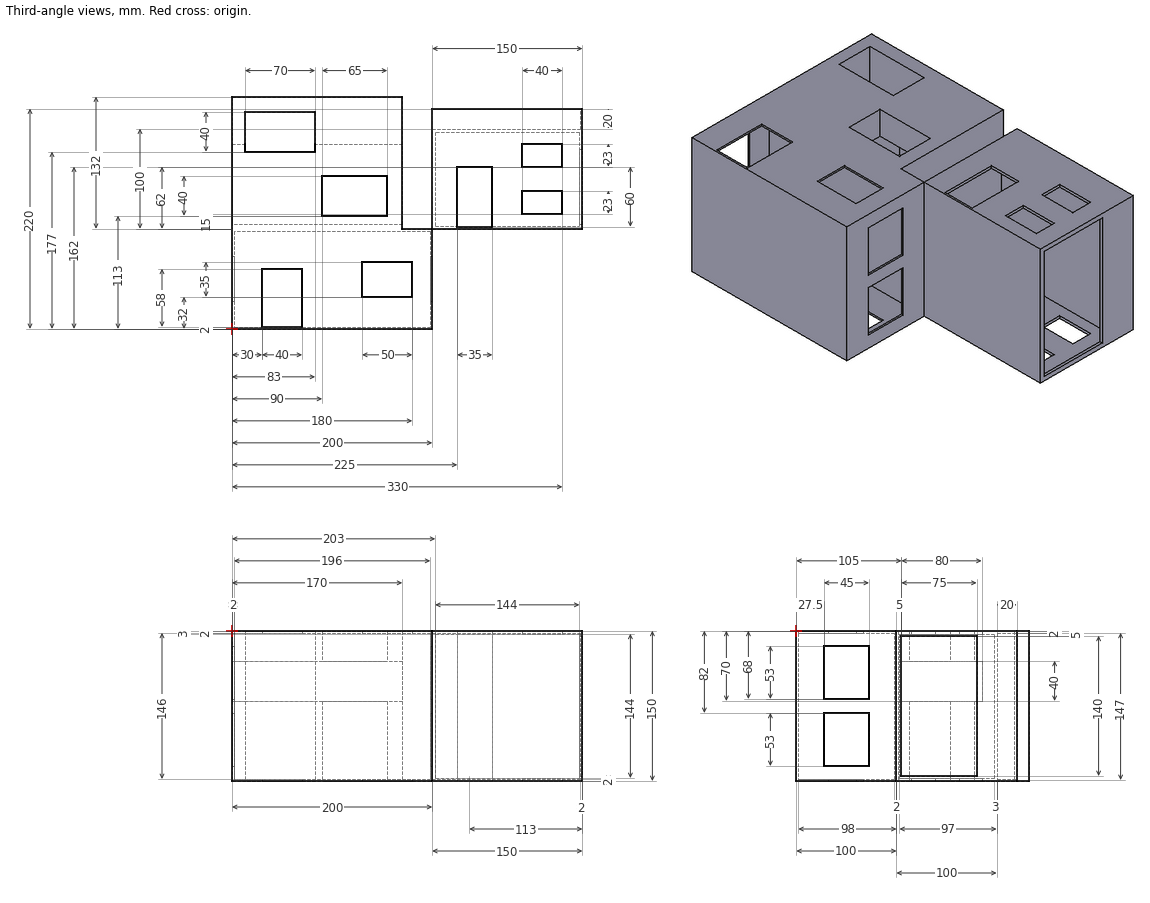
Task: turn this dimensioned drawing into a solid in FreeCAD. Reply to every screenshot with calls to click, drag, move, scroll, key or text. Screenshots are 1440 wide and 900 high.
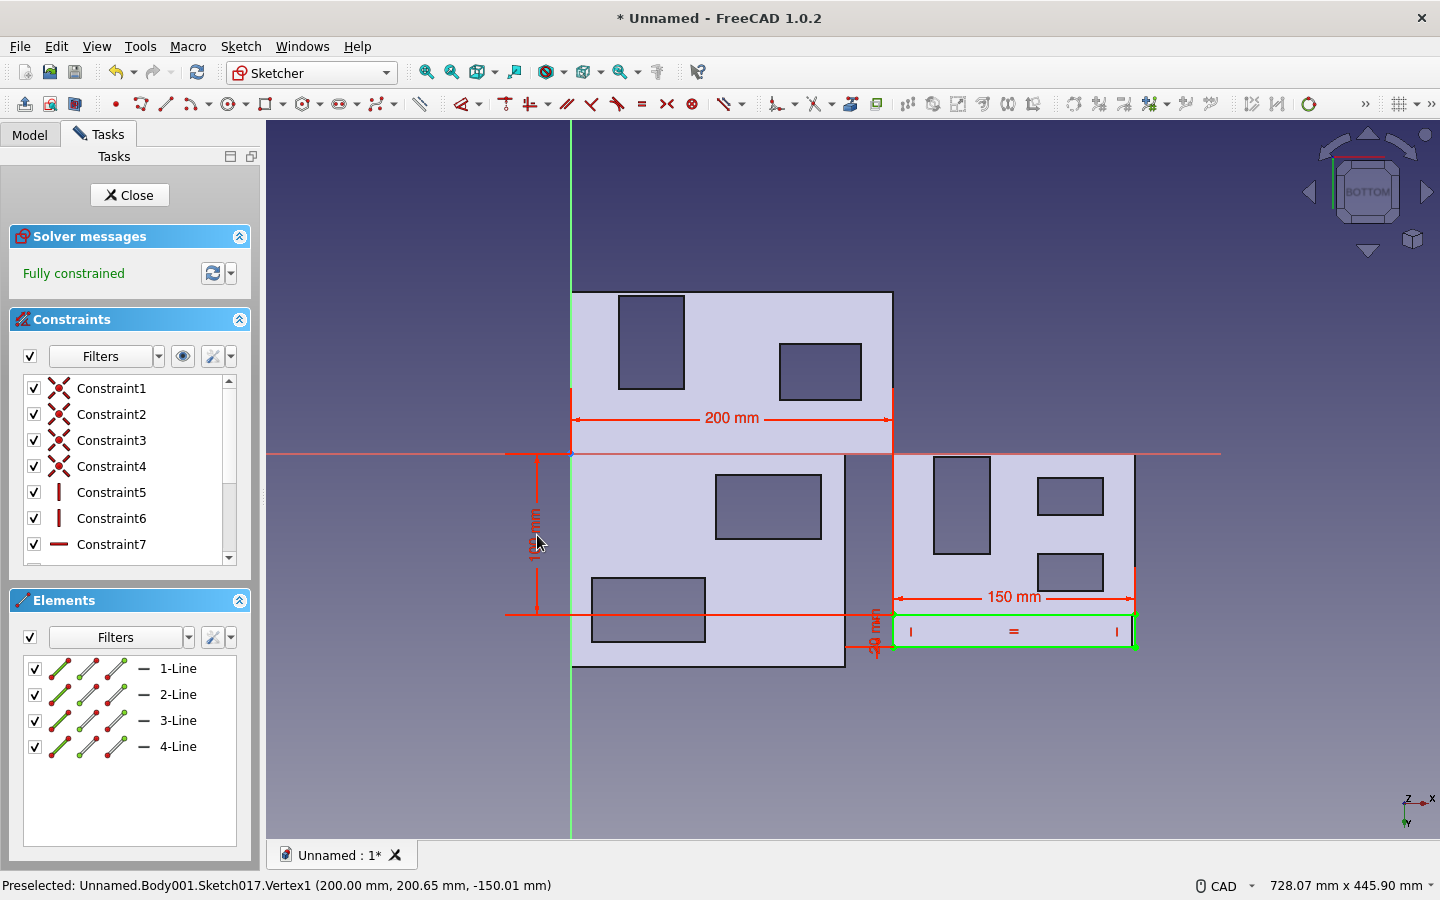
click(130, 195)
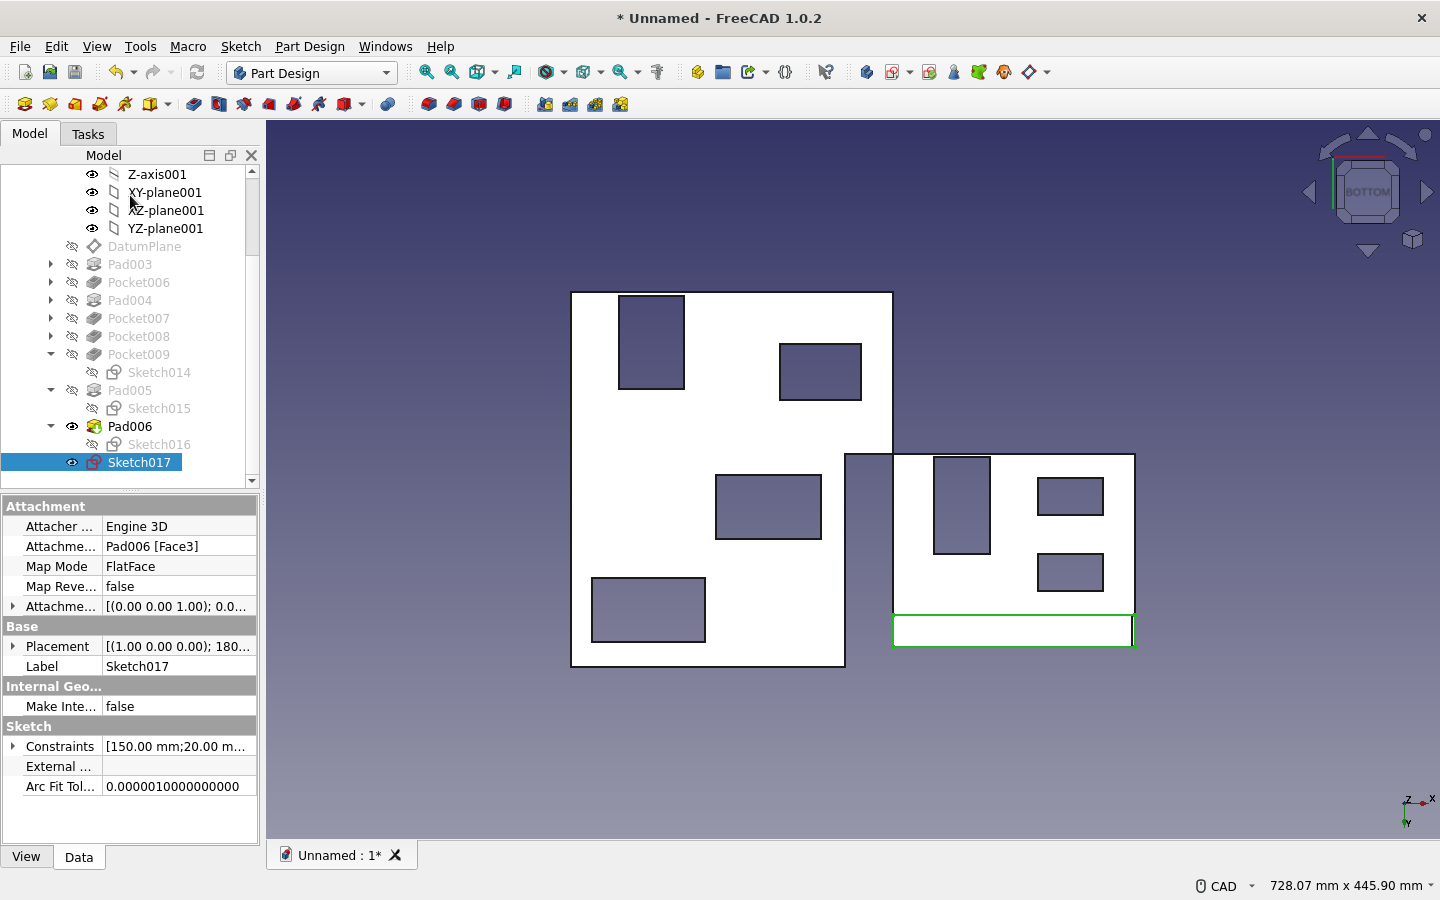
click(25, 104)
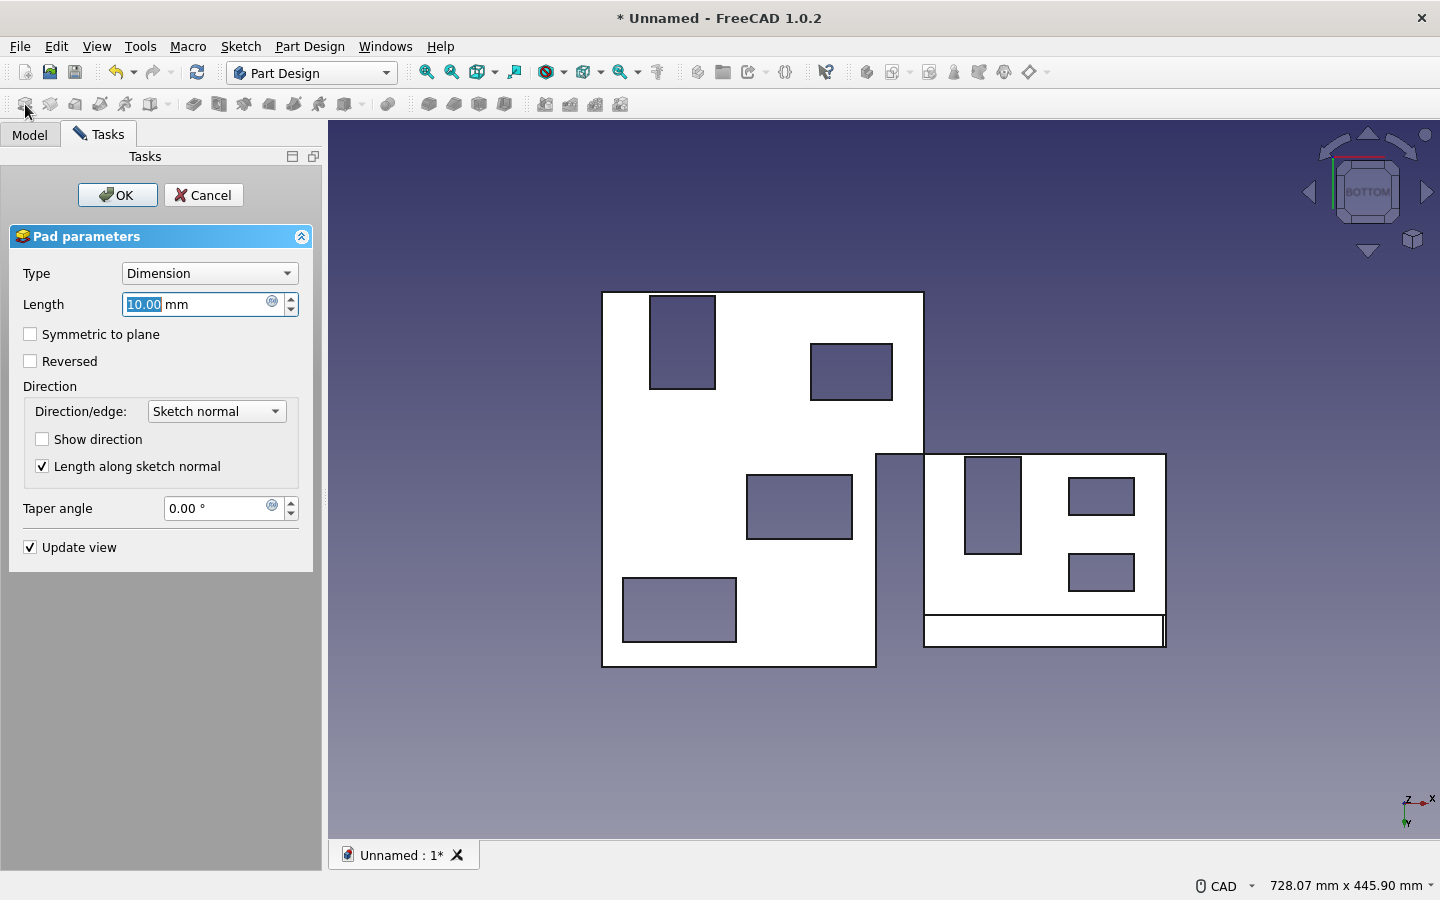
text(2)
key(Tab)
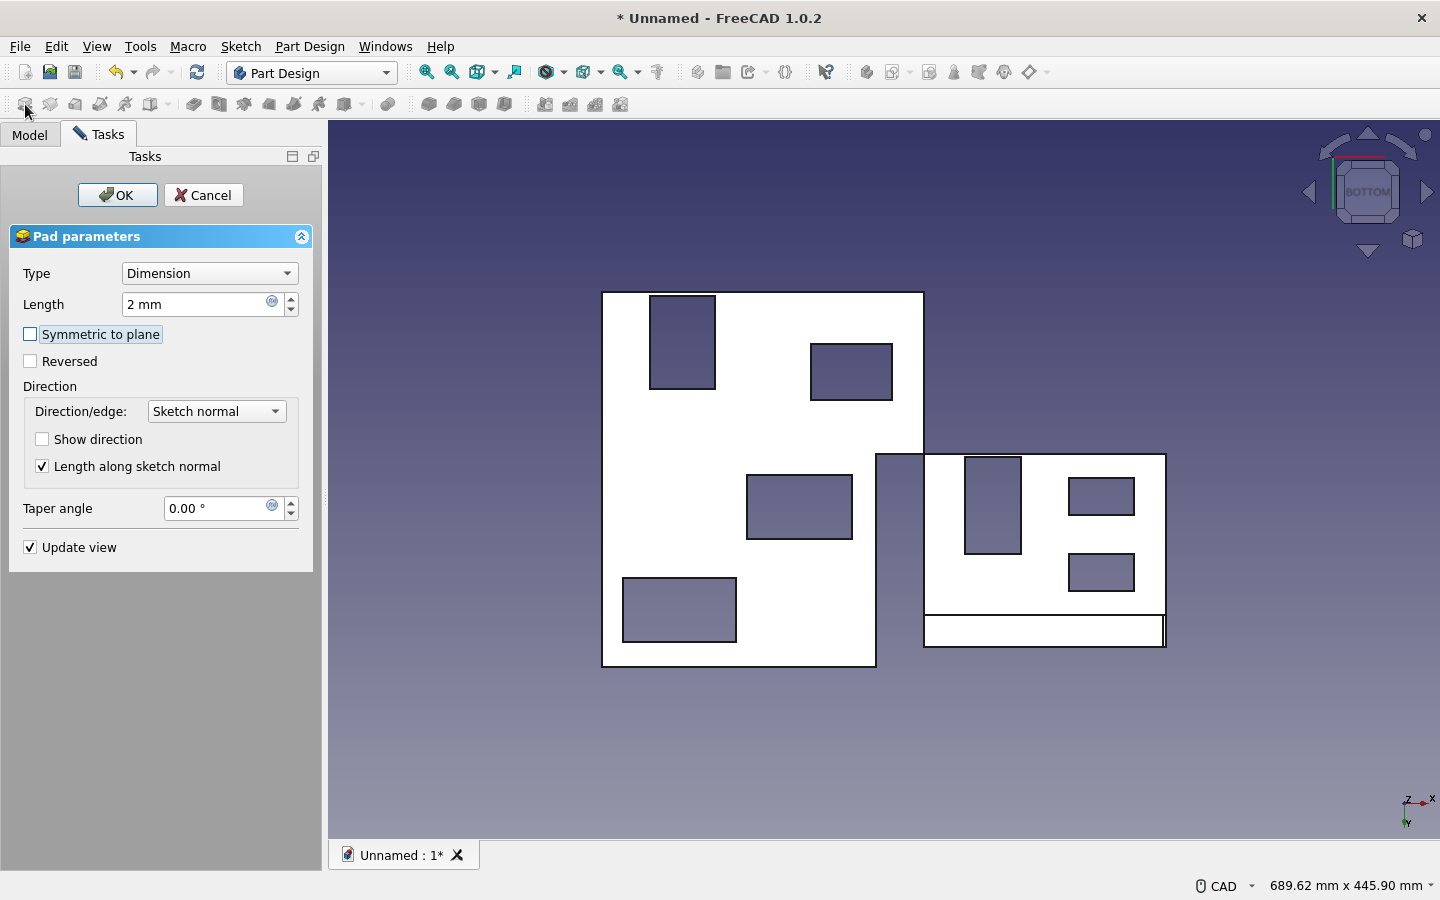
click(31, 361)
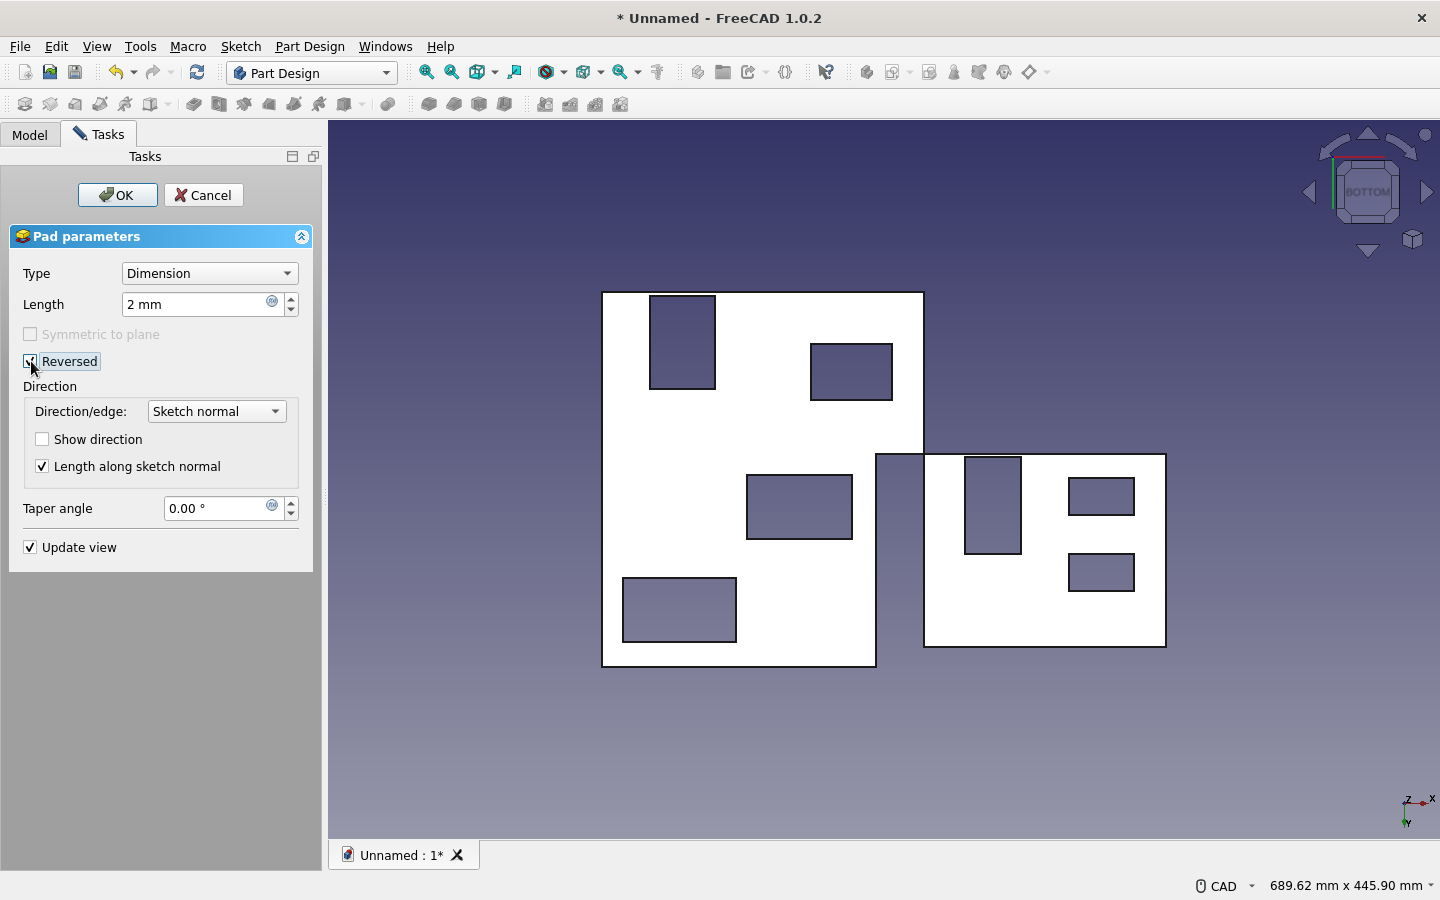
click(118, 195)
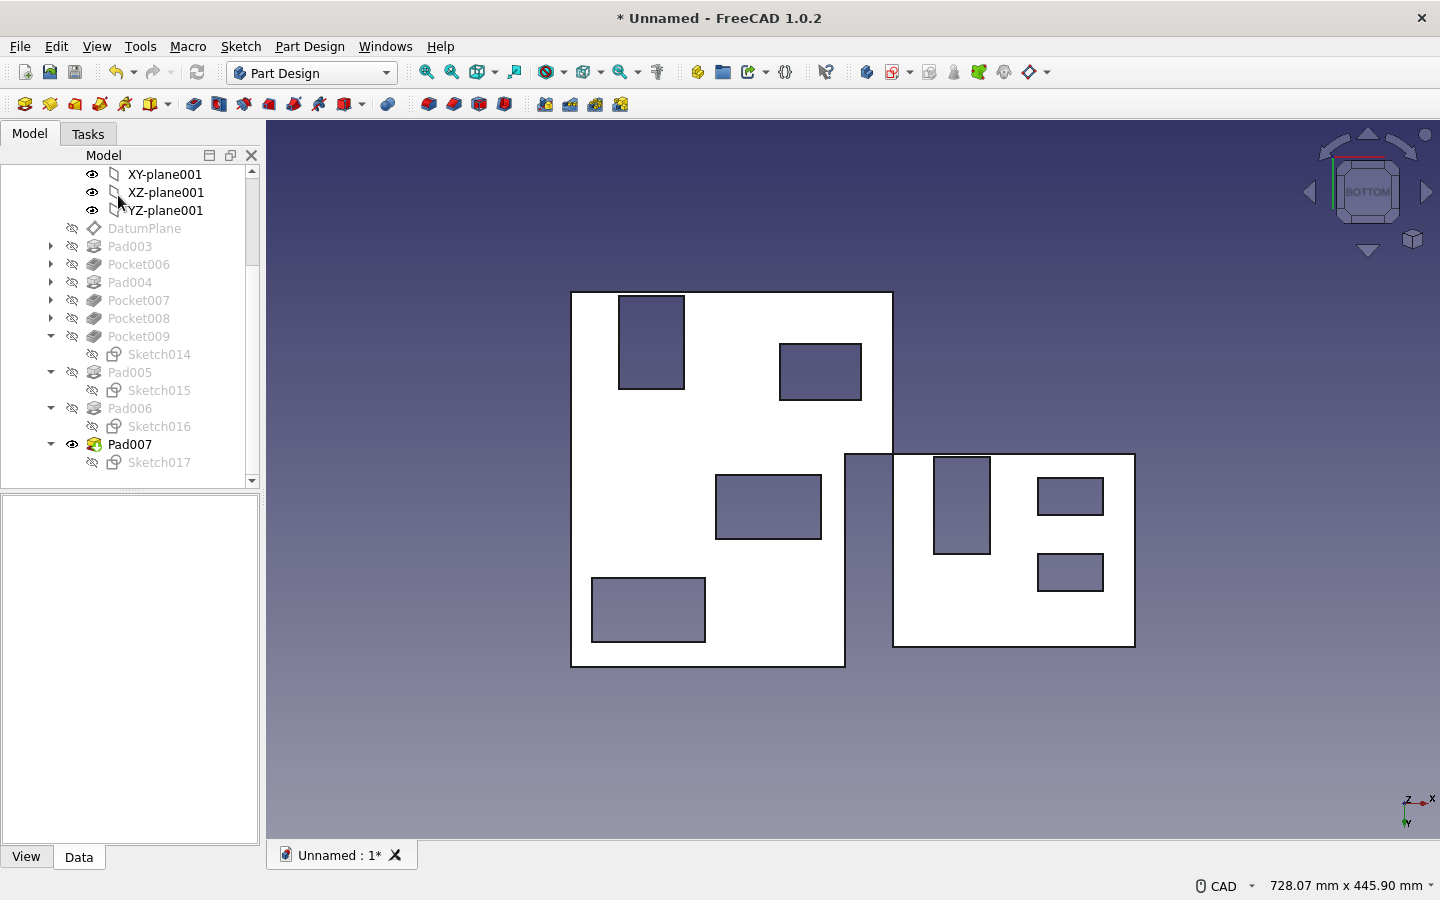
key(0)